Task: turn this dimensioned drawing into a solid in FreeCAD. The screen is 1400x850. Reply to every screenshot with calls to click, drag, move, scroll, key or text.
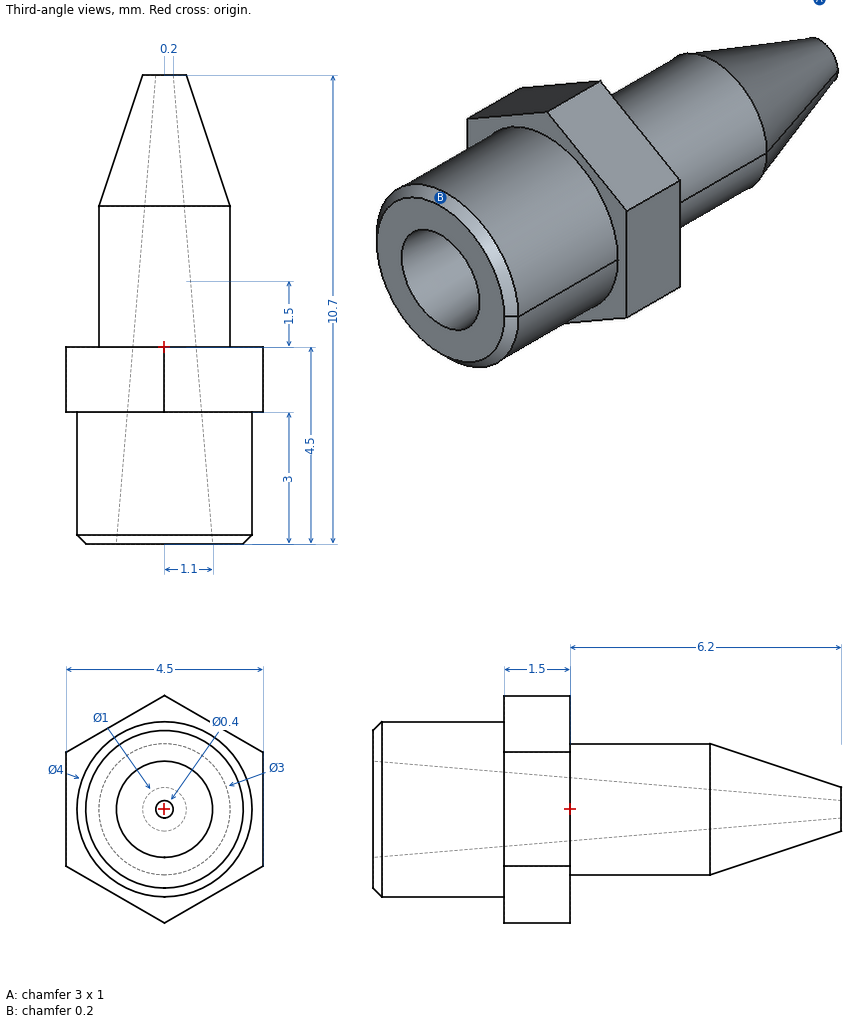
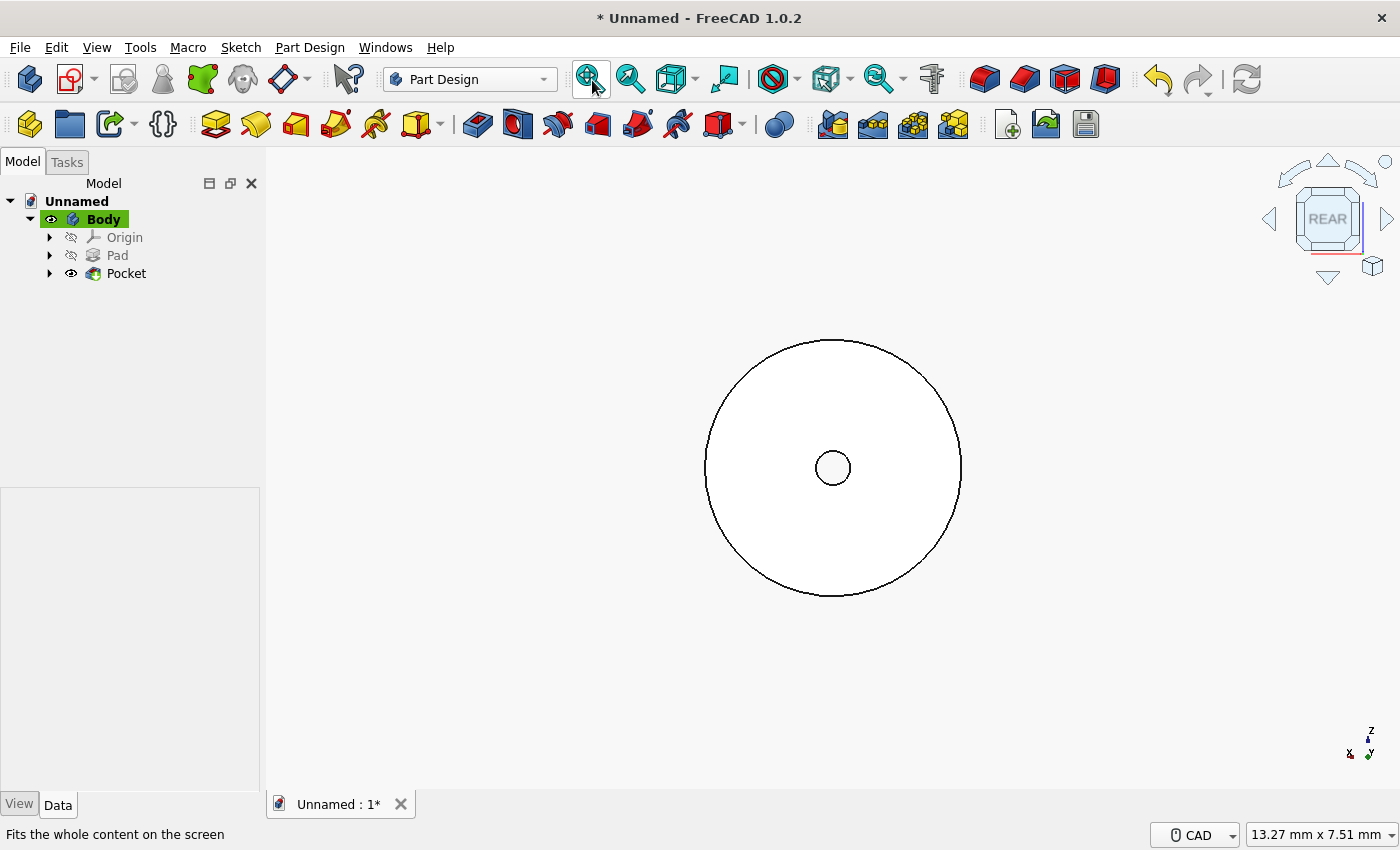
click(961, 467)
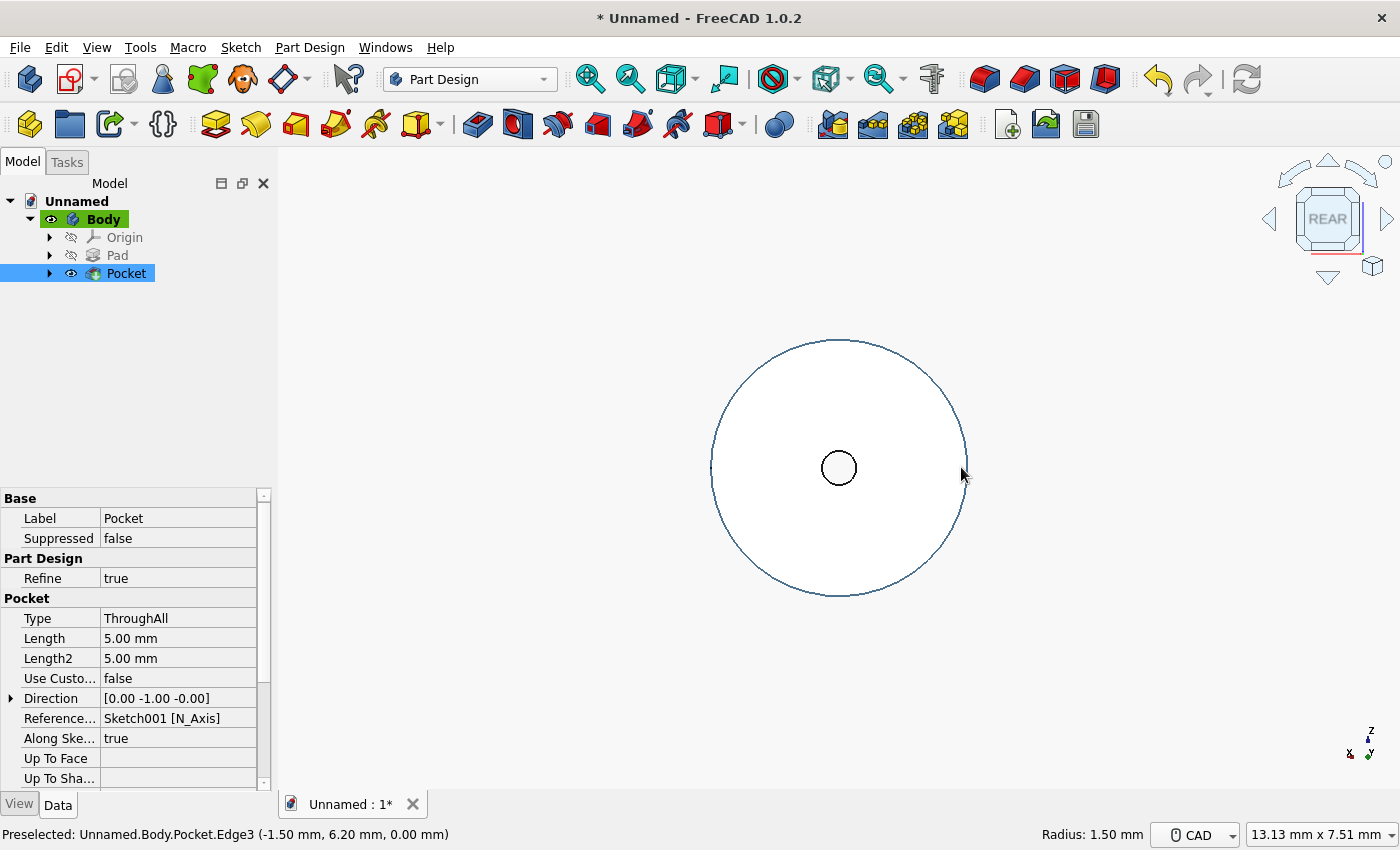
click(1026, 80)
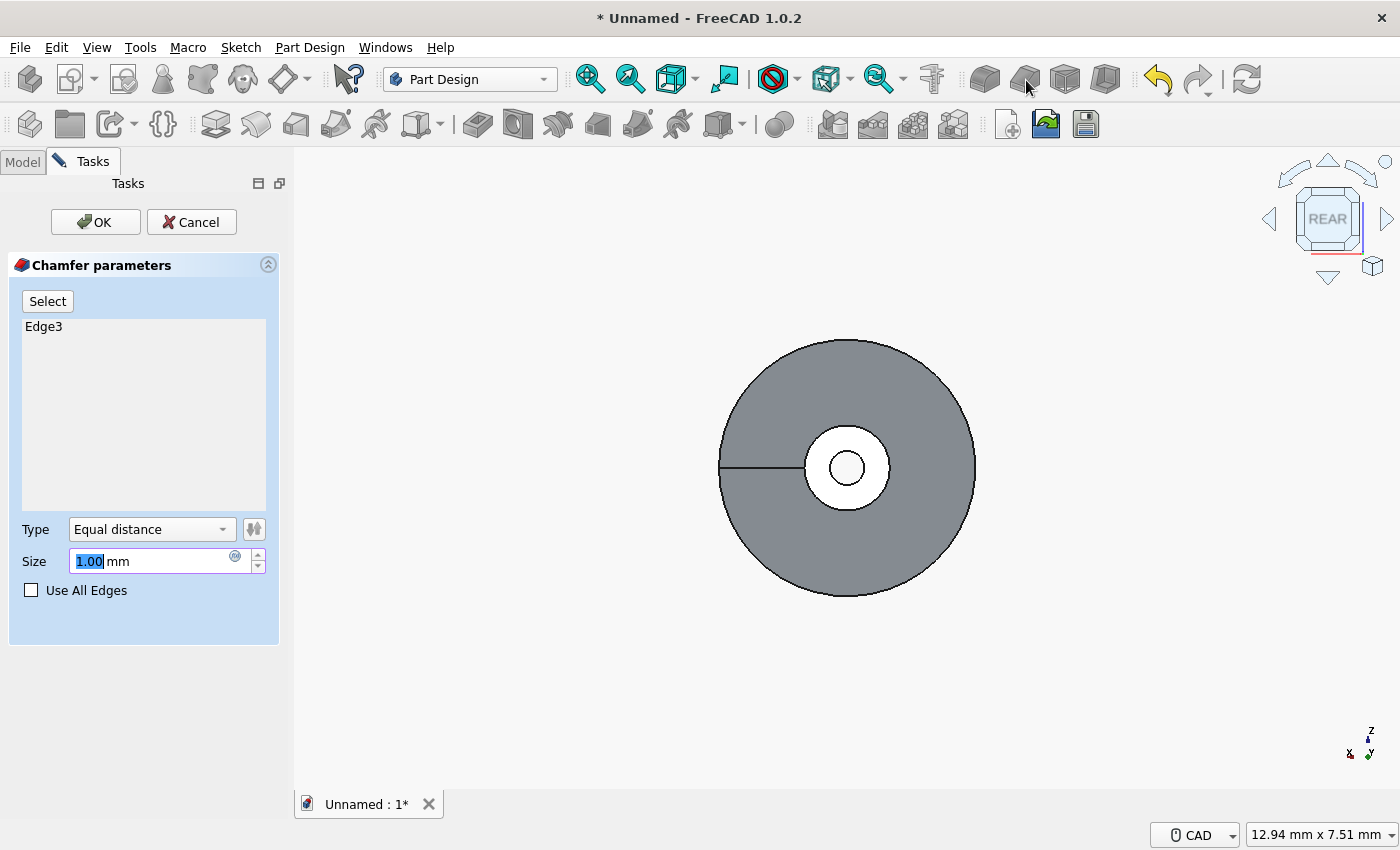
text(3)
key(Tab)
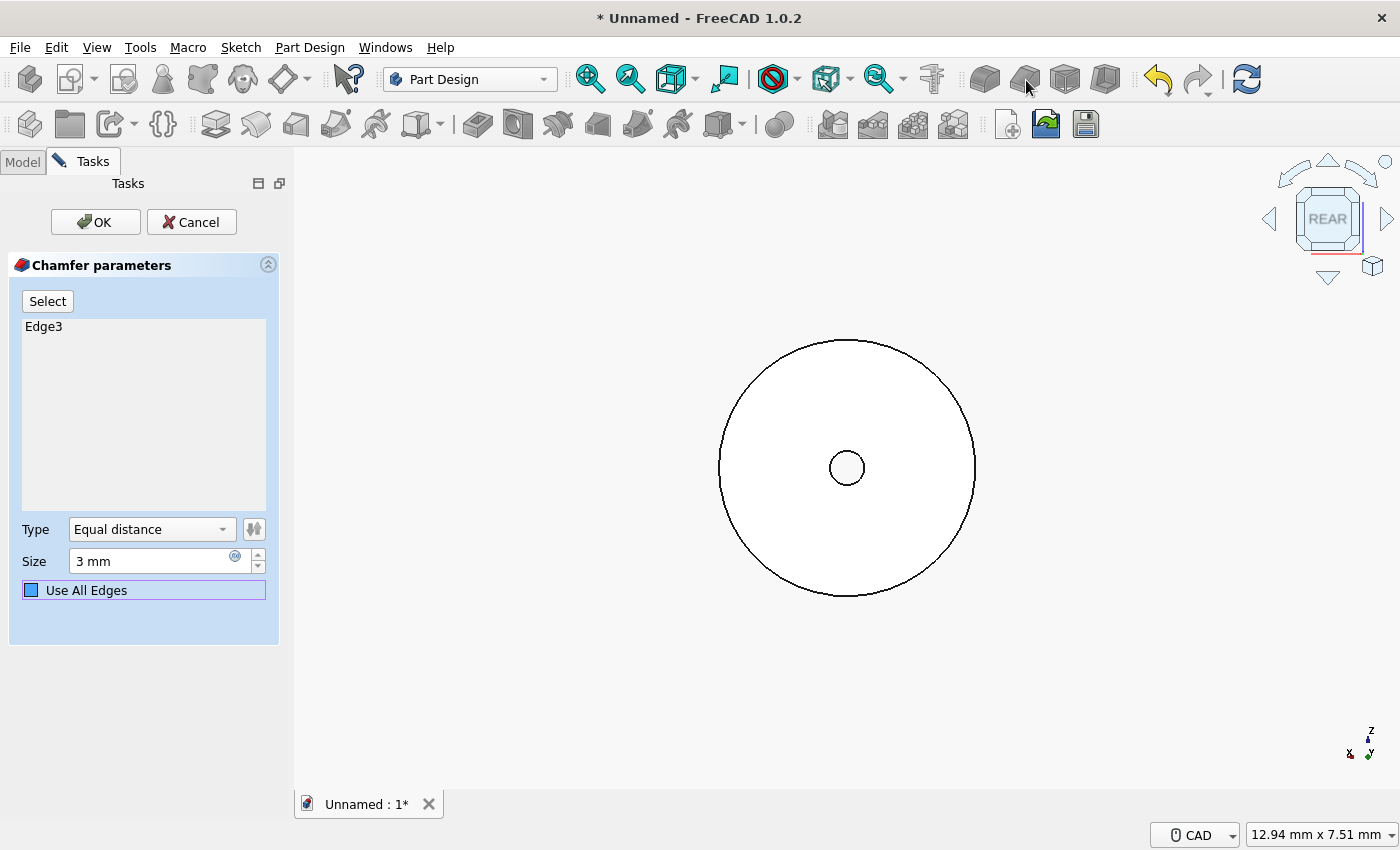
click(153, 530)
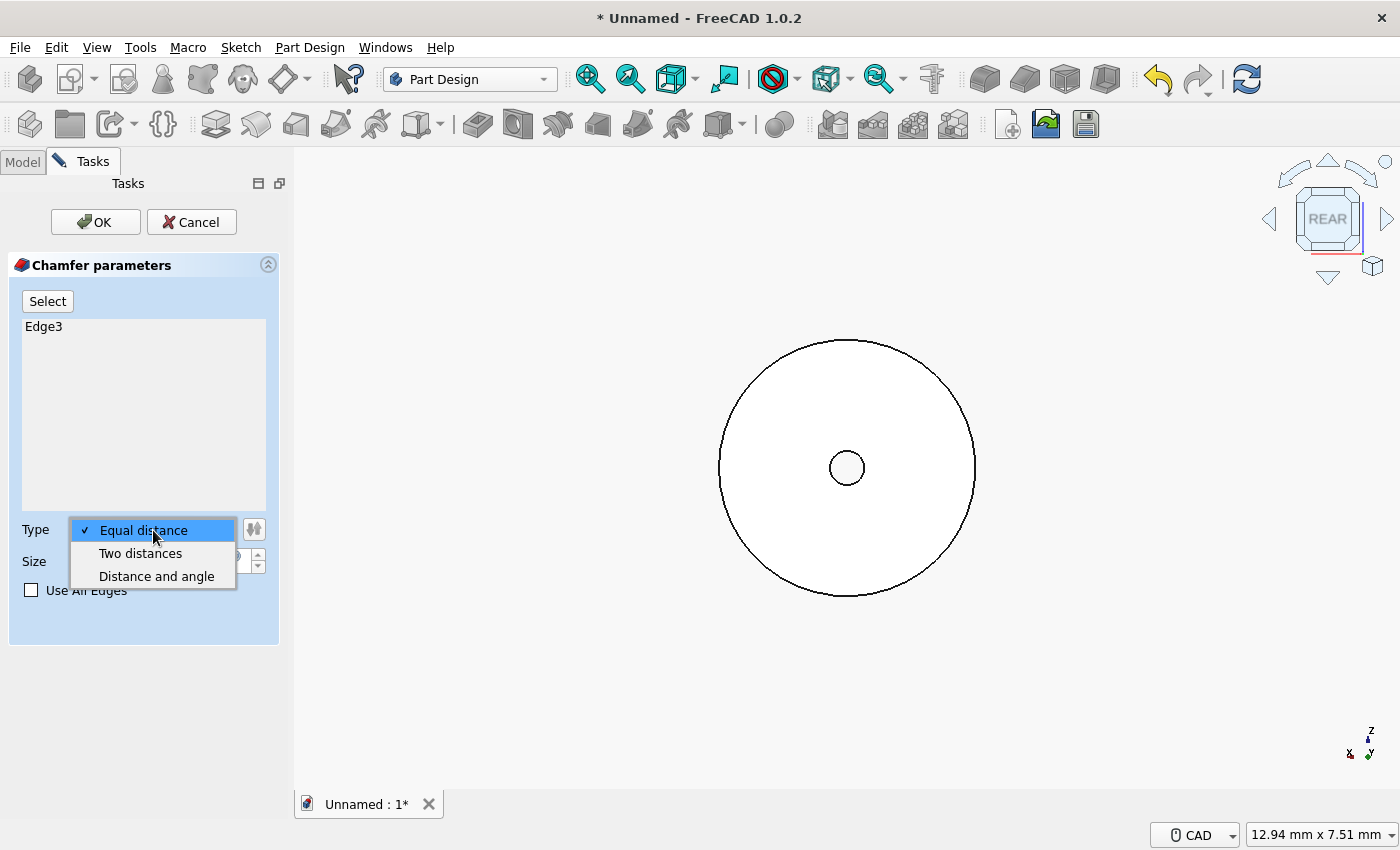
click(152, 554)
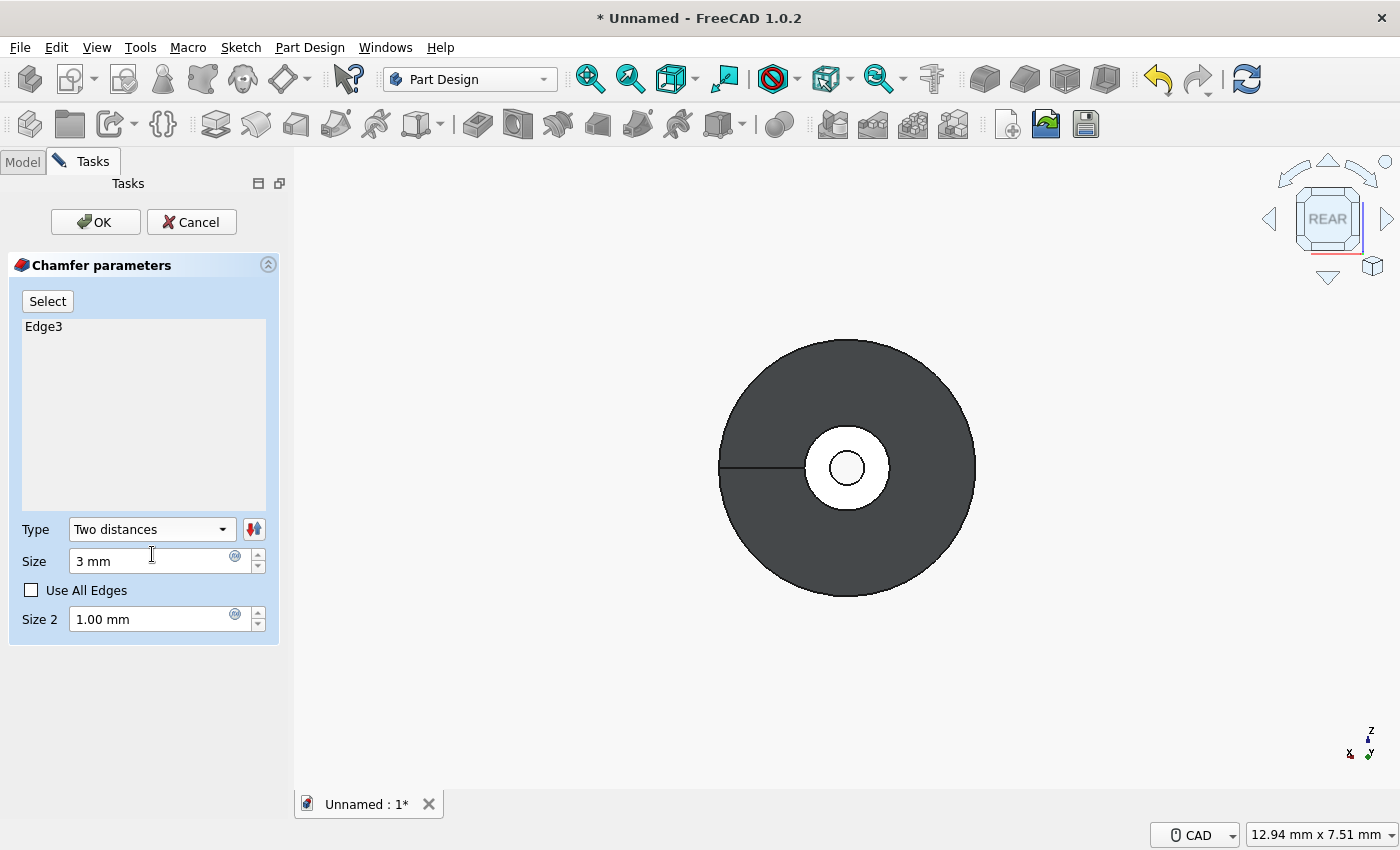
triple_click(160, 619)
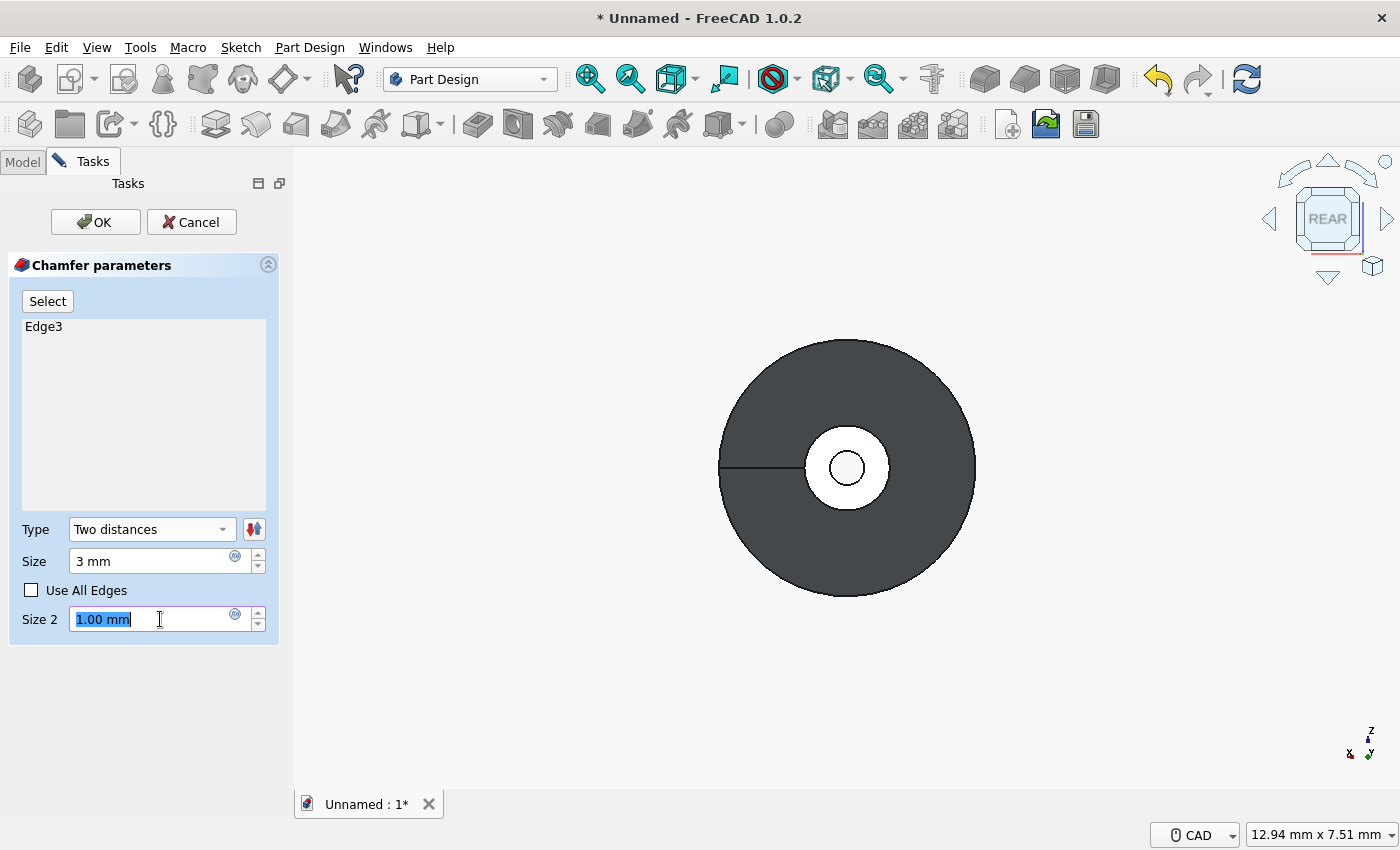
text(1)
key(Tab)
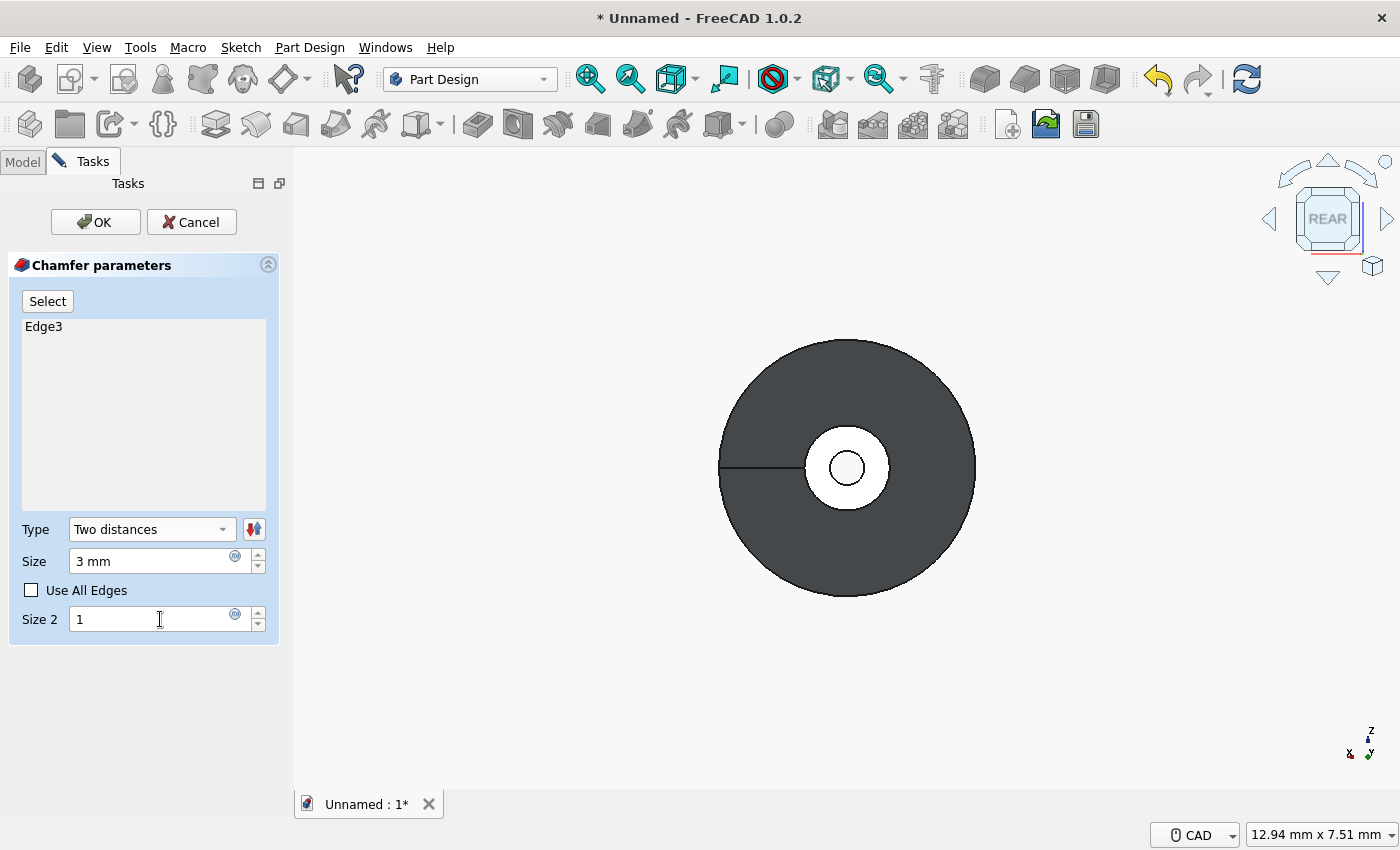
click(96, 222)